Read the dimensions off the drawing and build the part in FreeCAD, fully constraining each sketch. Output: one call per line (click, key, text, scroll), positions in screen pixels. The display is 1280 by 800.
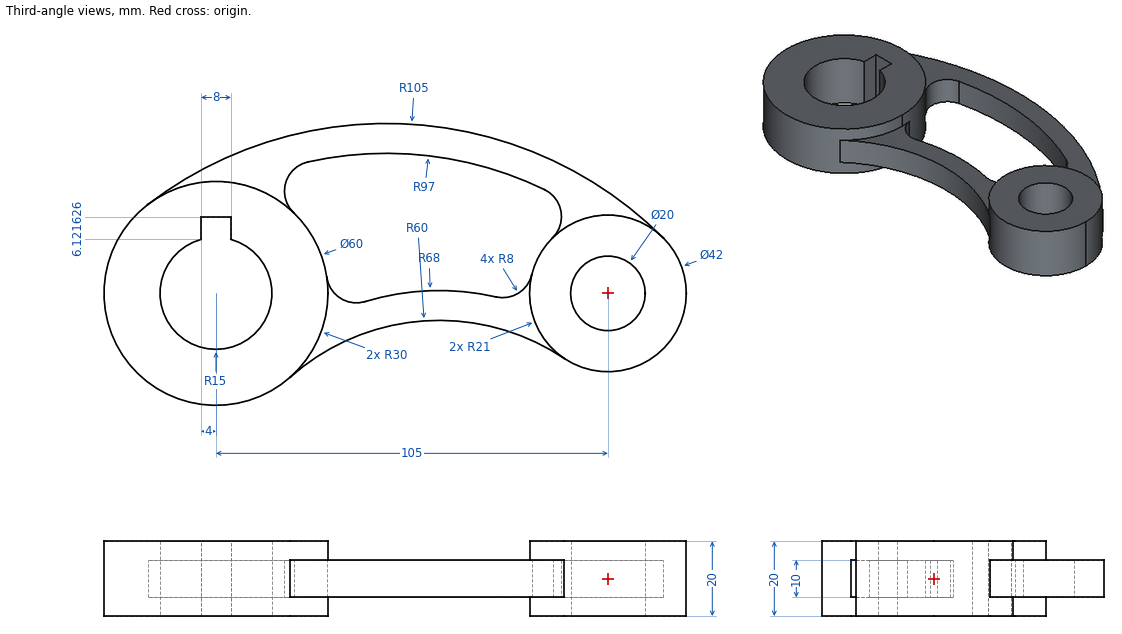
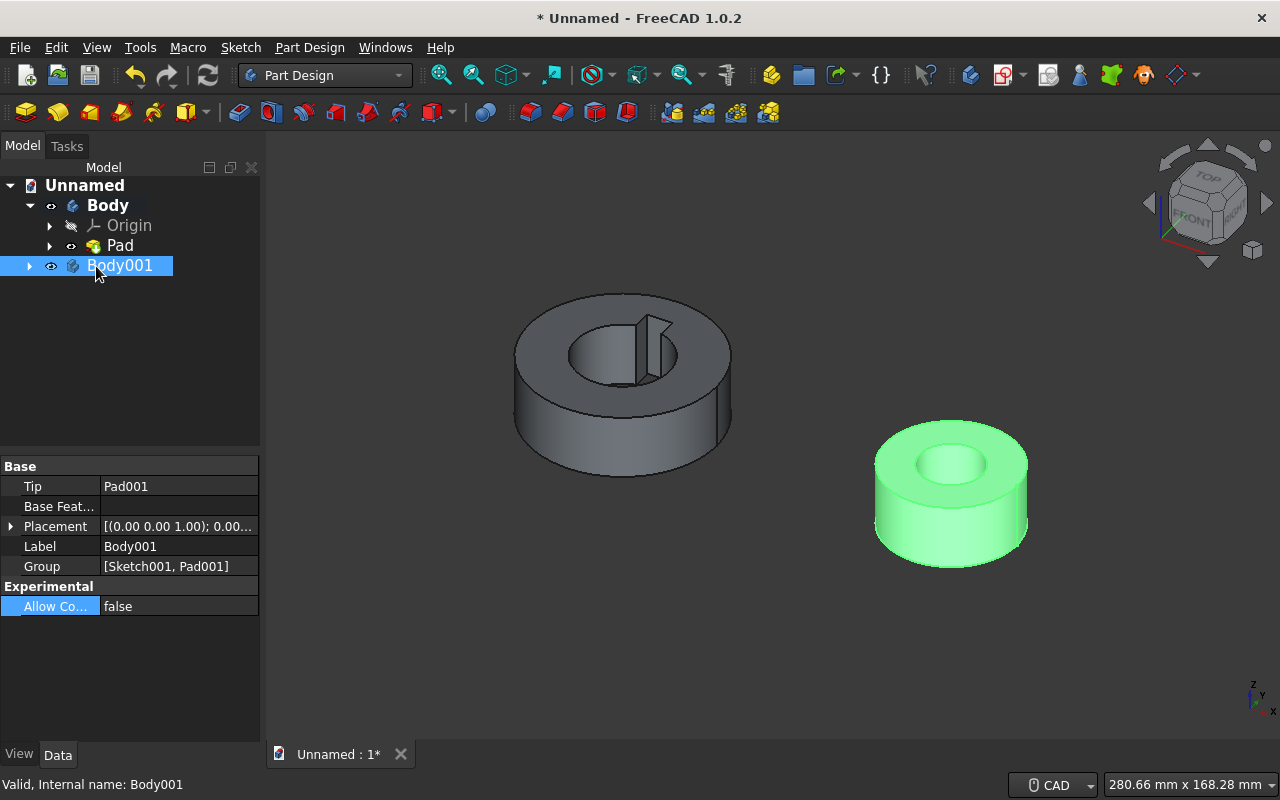
click(486, 112)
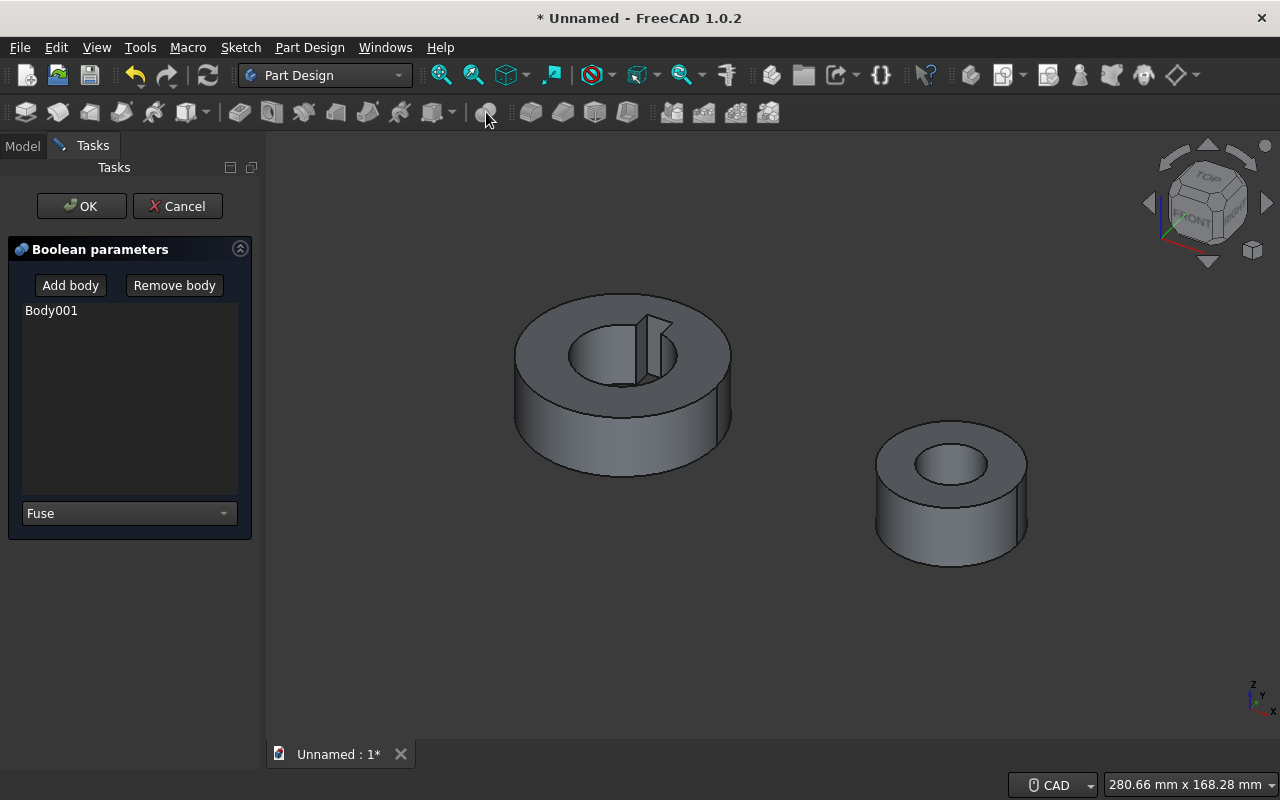
click(82, 206)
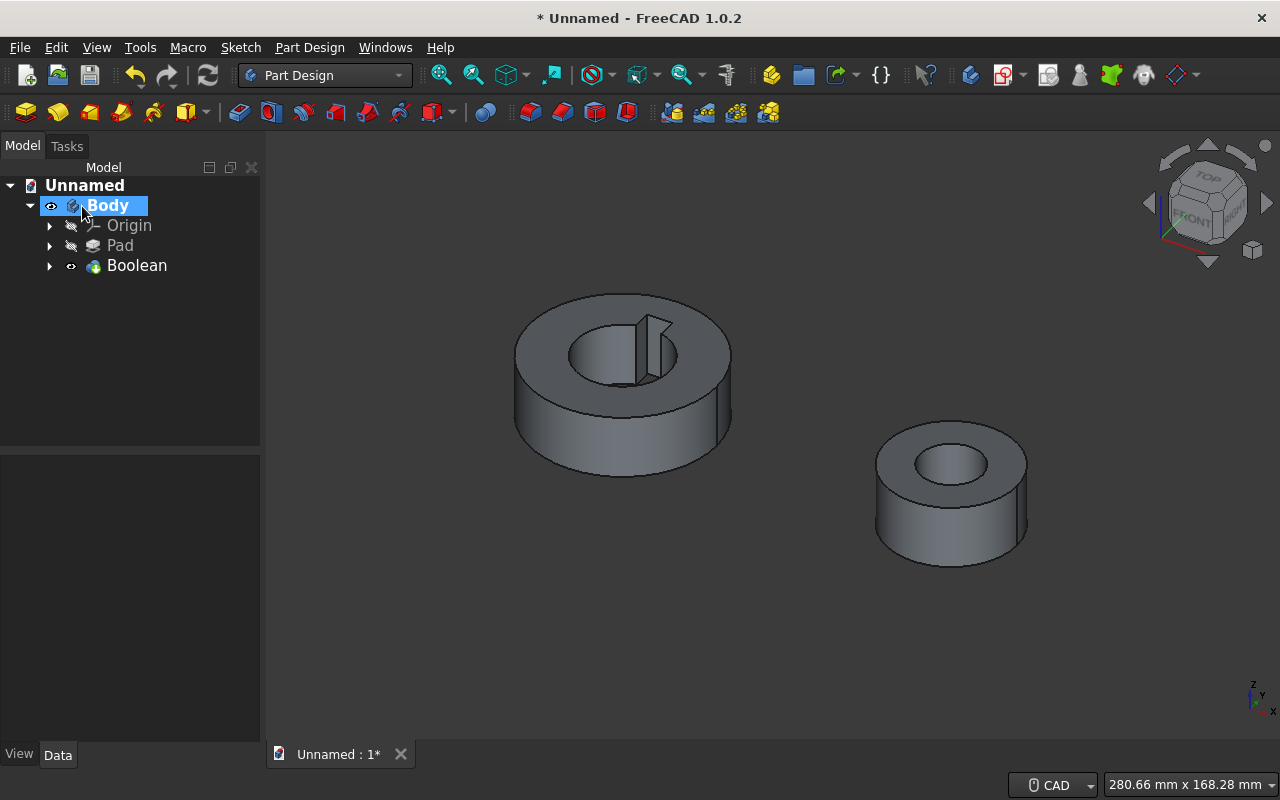
click(1004, 76)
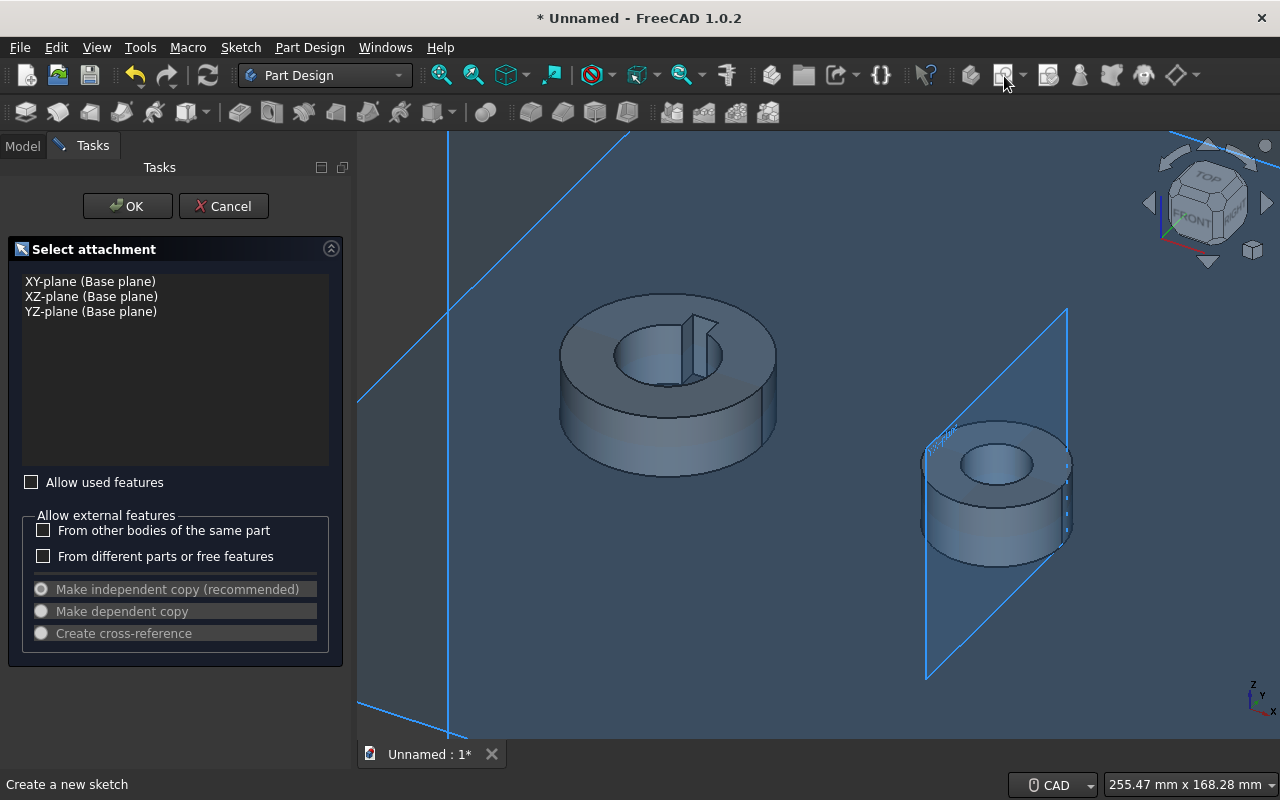
click(82, 282)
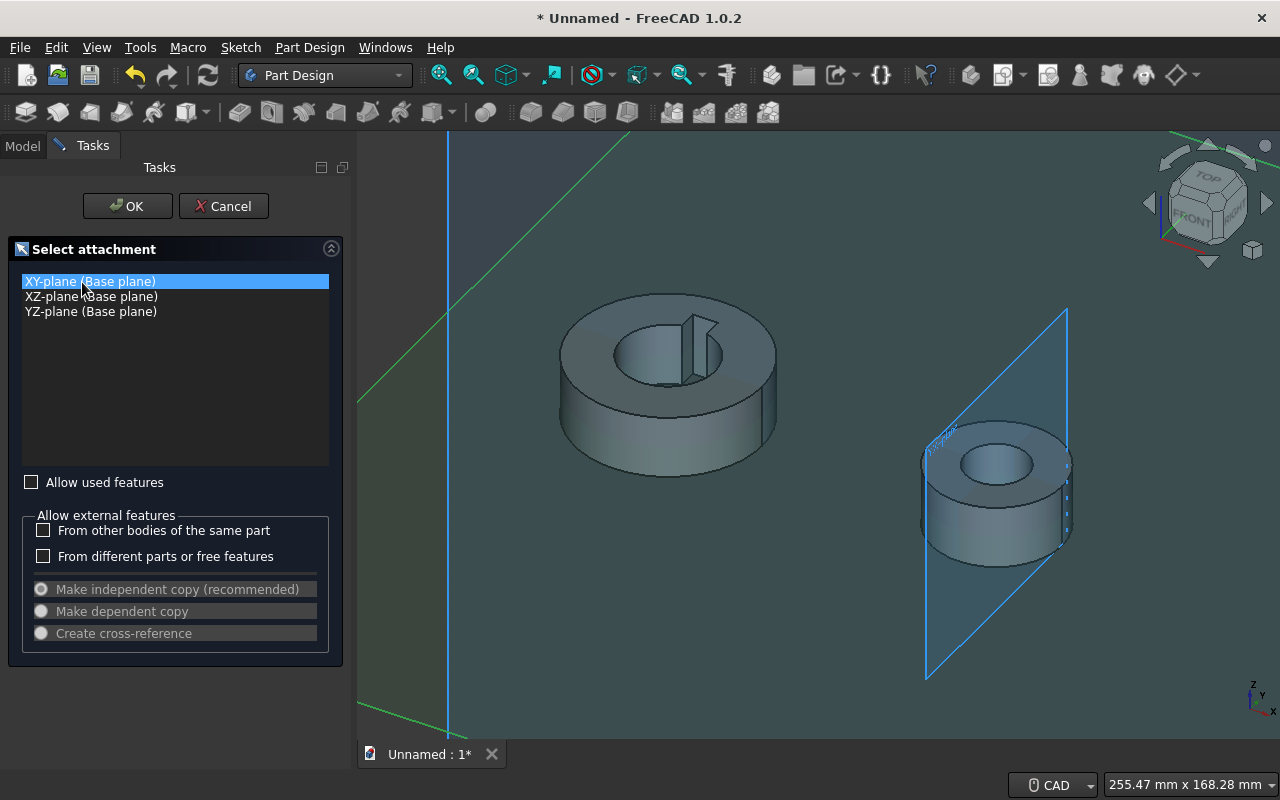
click(128, 206)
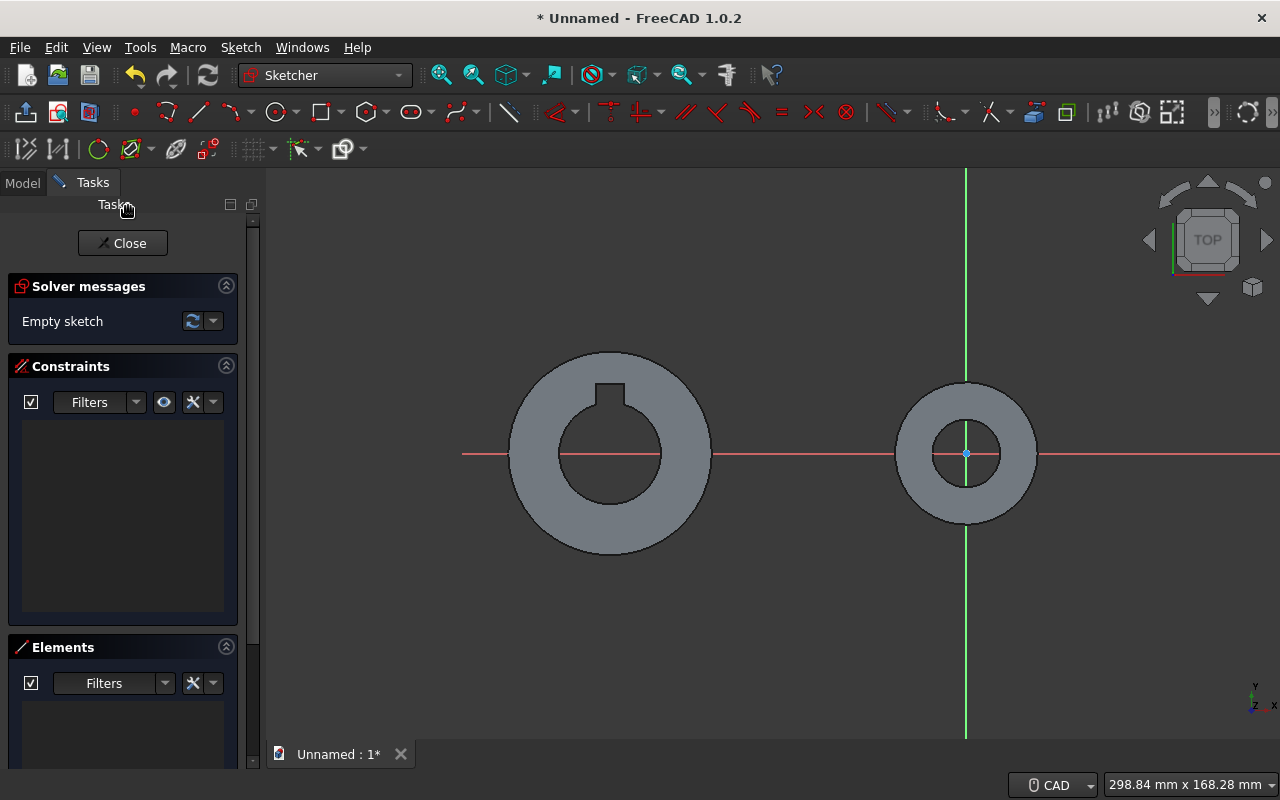
key(q)
key(s)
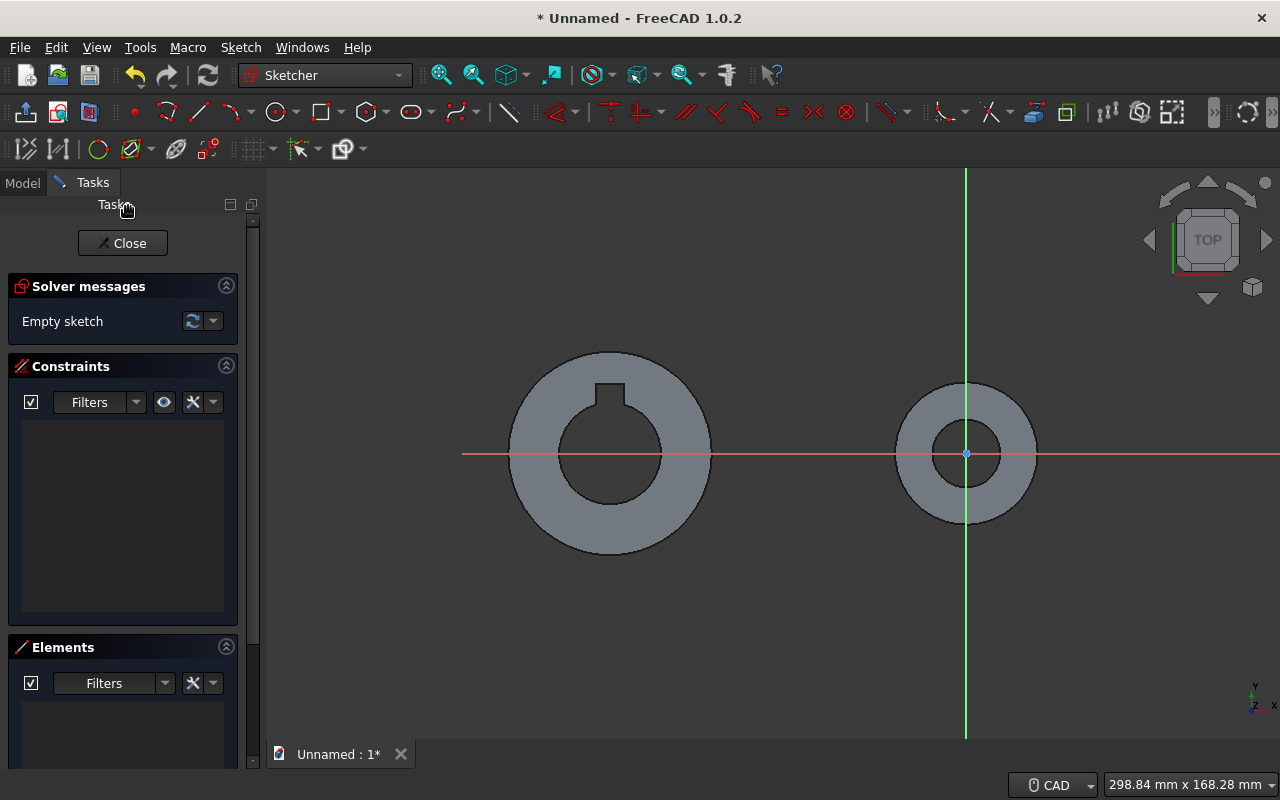
key(g)
key(3)
key(a)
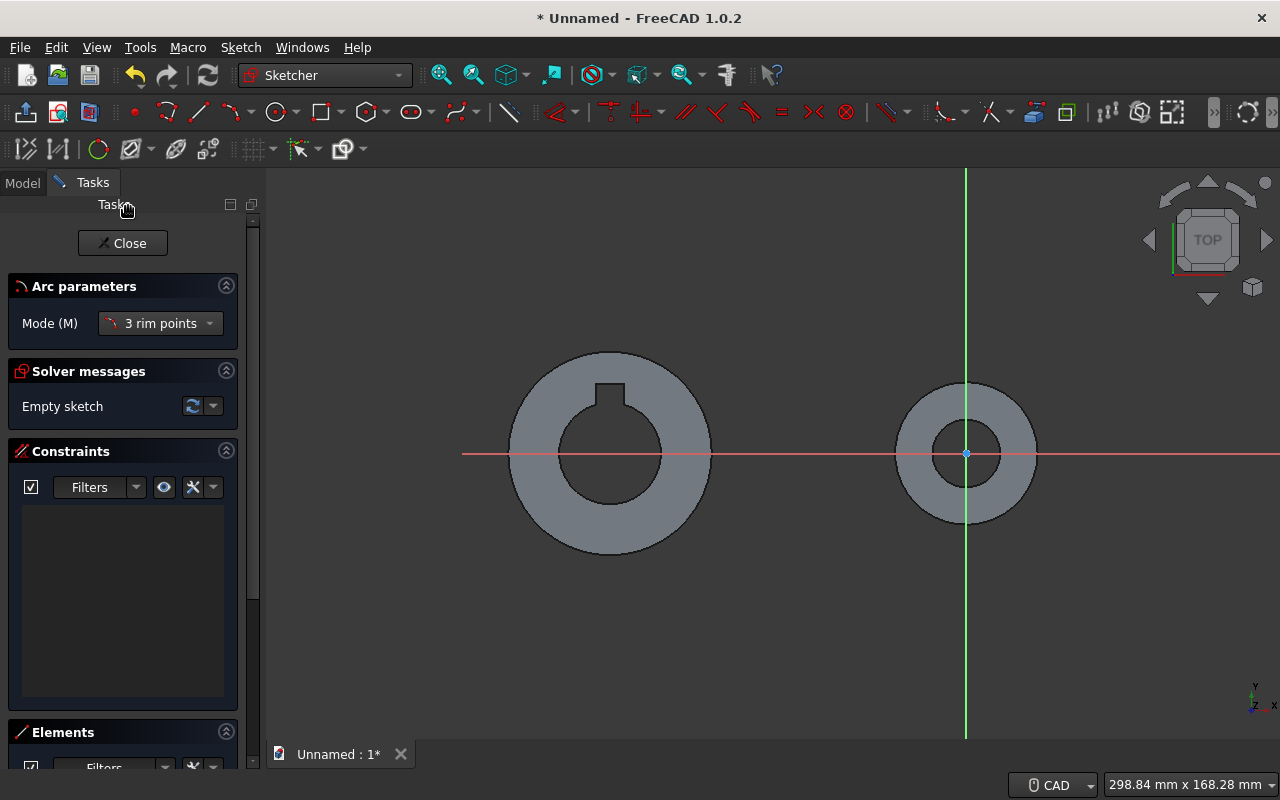
click(927, 513)
click(897, 437)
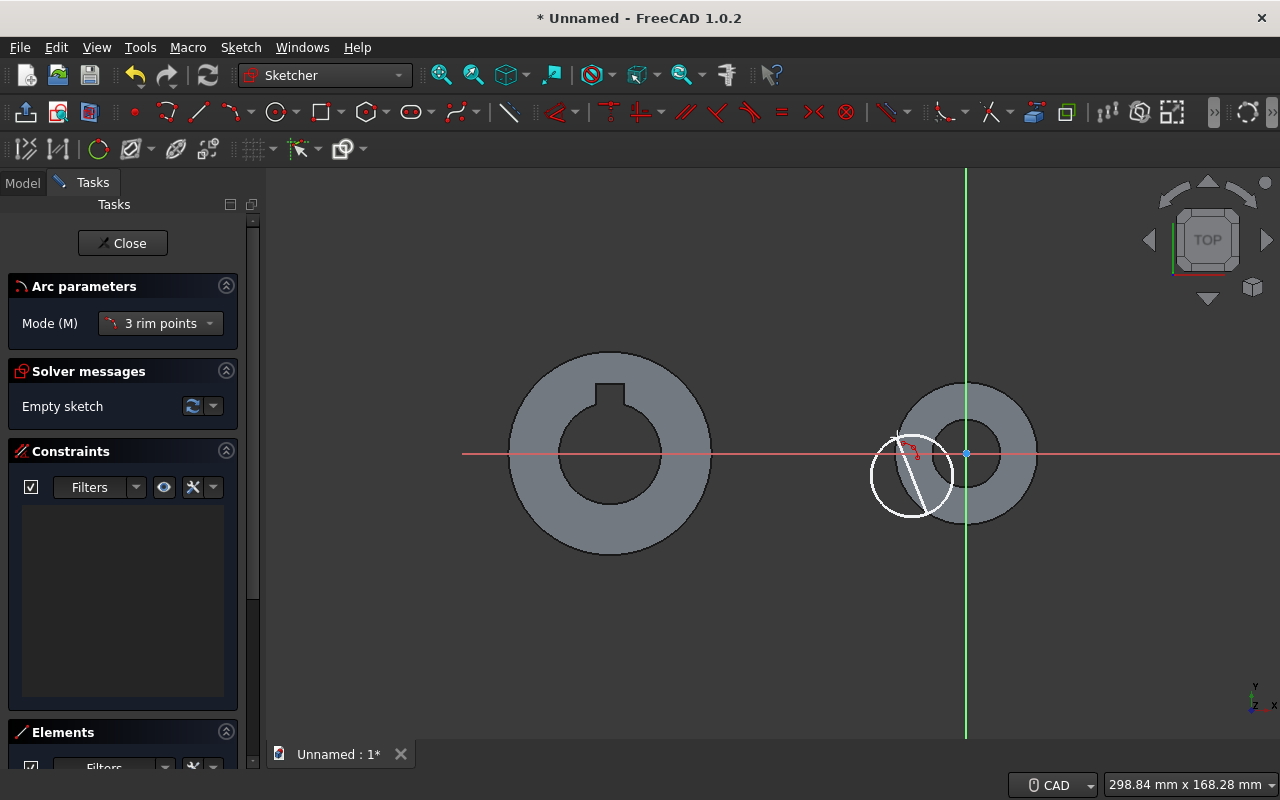
scroll(900, 479, up, 2)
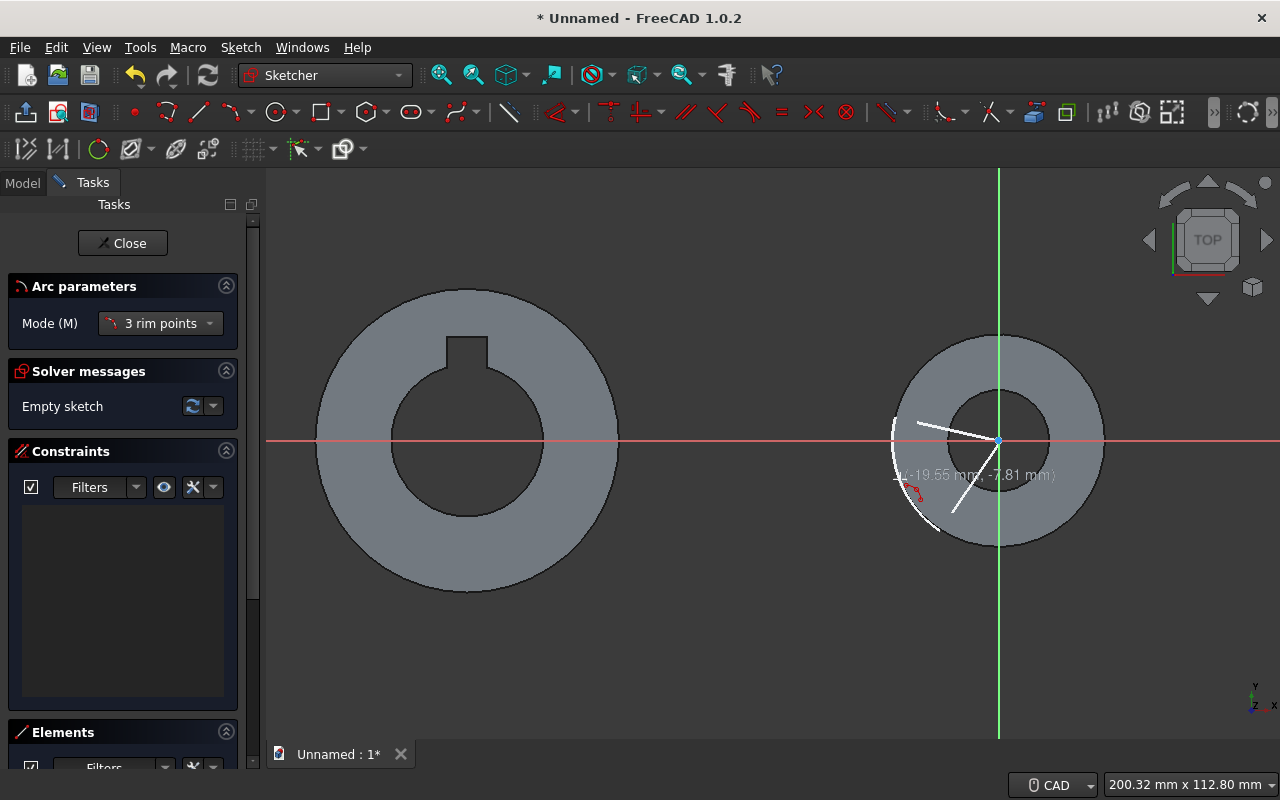
click(900, 479)